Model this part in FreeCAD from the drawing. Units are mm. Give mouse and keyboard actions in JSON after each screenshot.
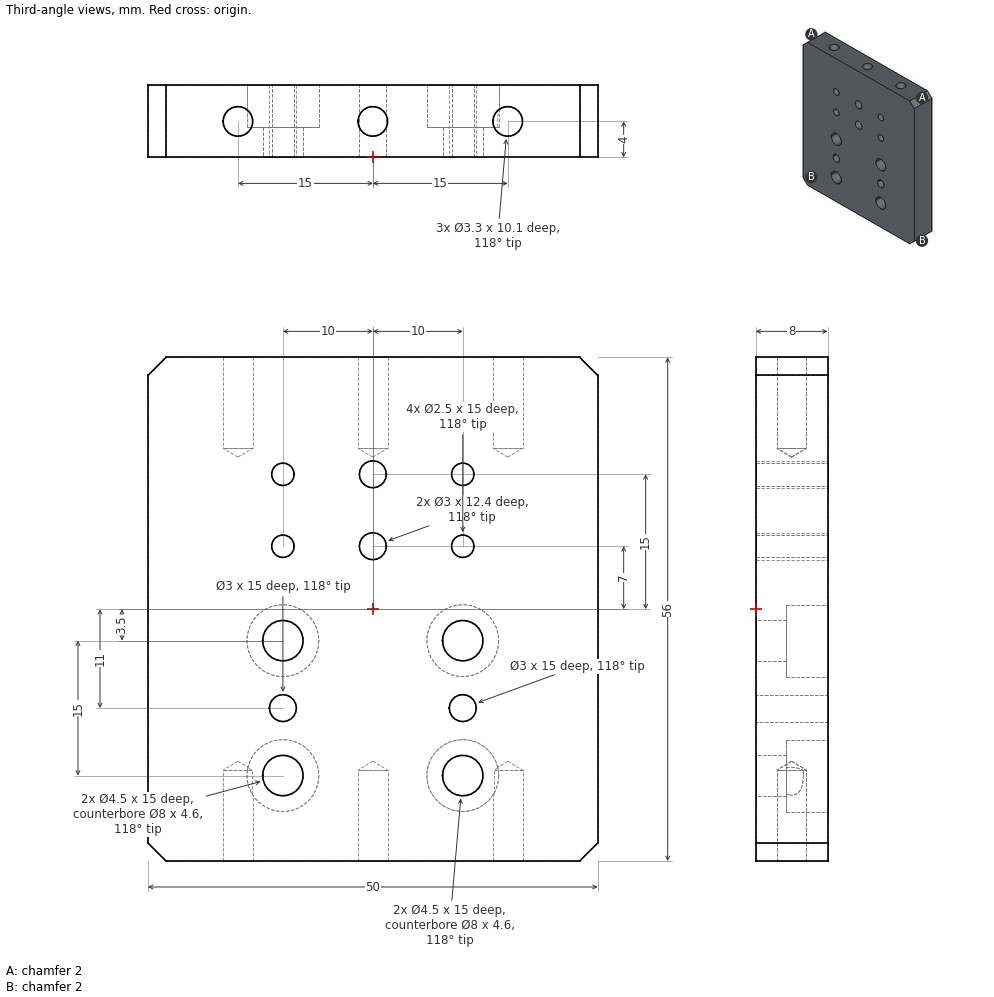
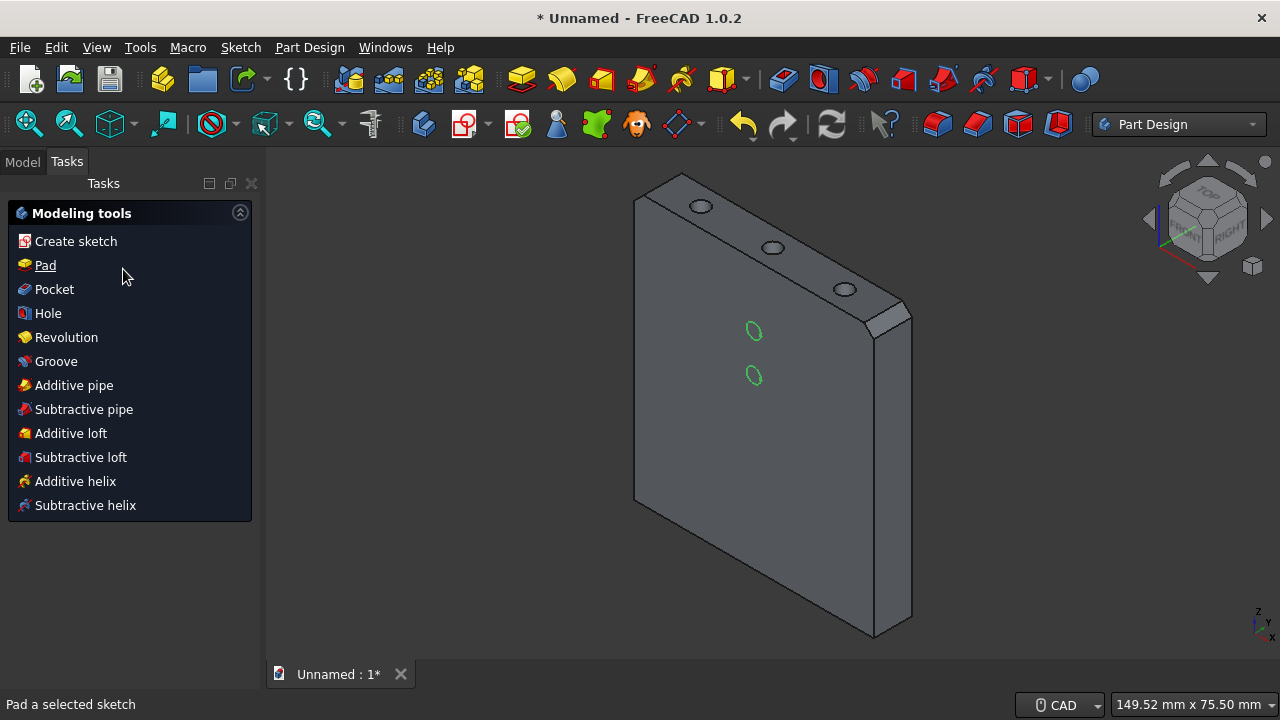
{"action": "left_click", "coordinate": [824, 80]}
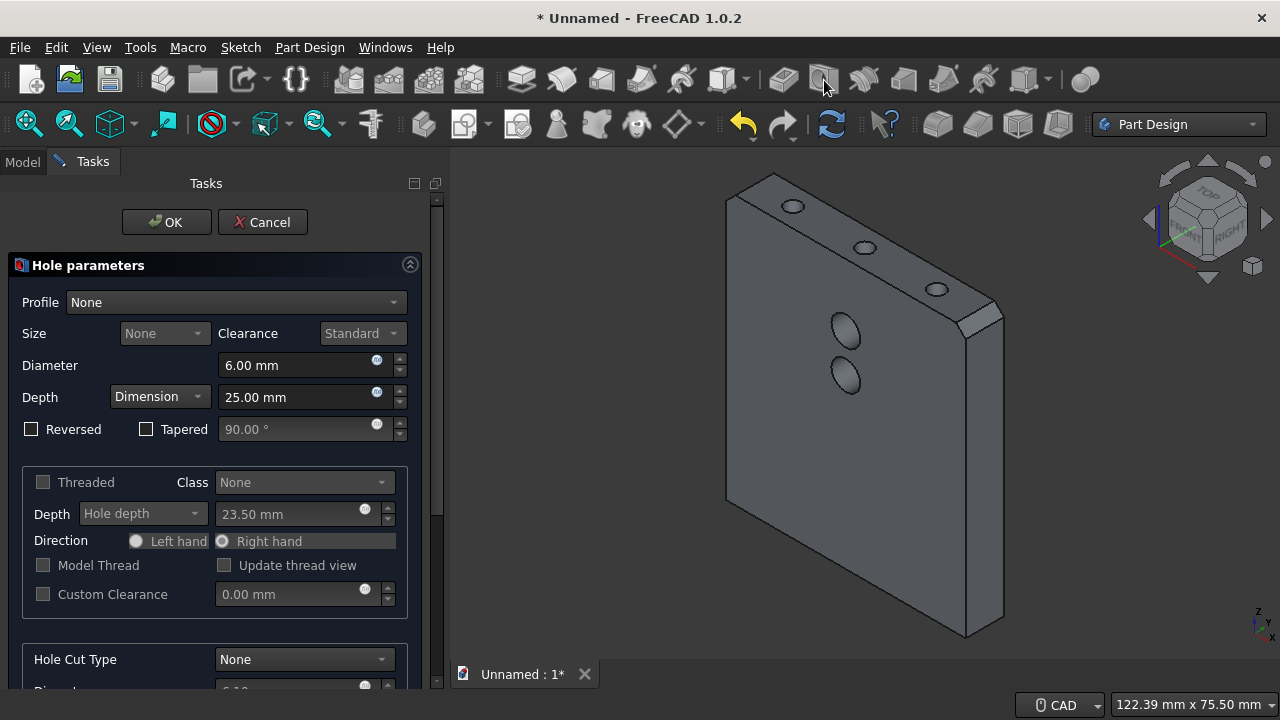
{"action": "triple_click", "coordinate": [305, 365]}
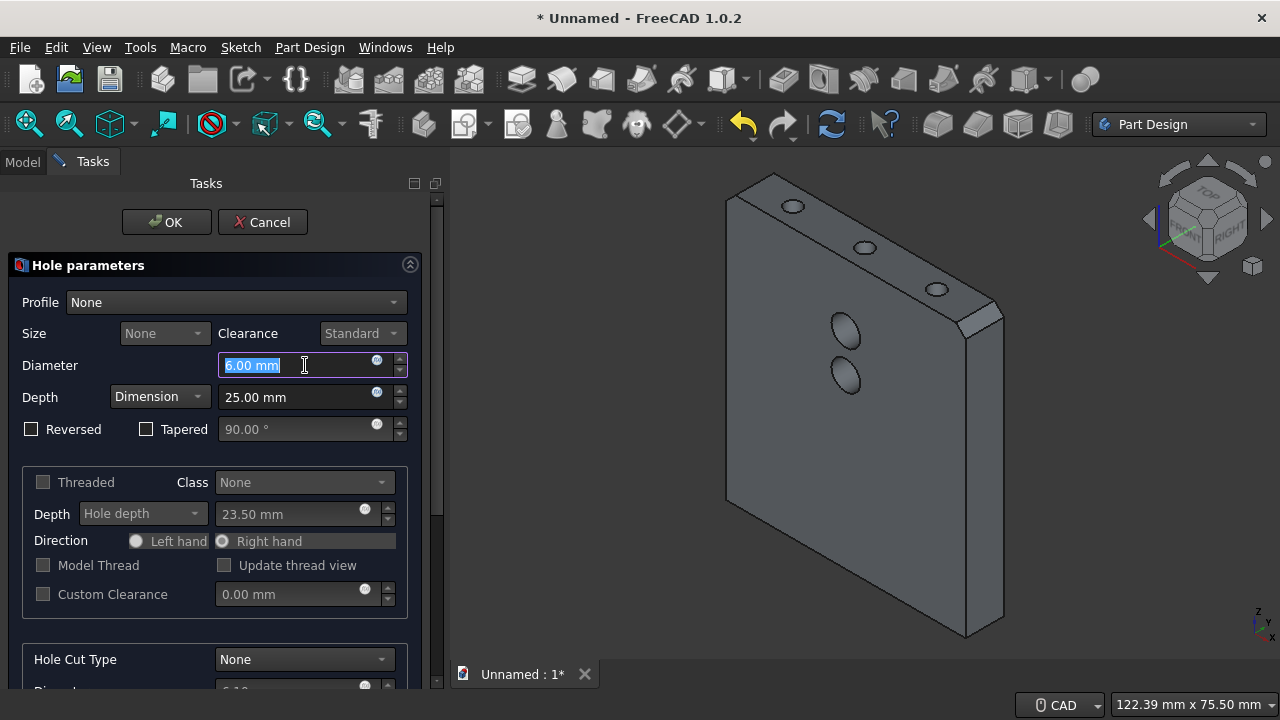
{"action": "type", "text": "3"}
{"action": "key", "text": "Tab"}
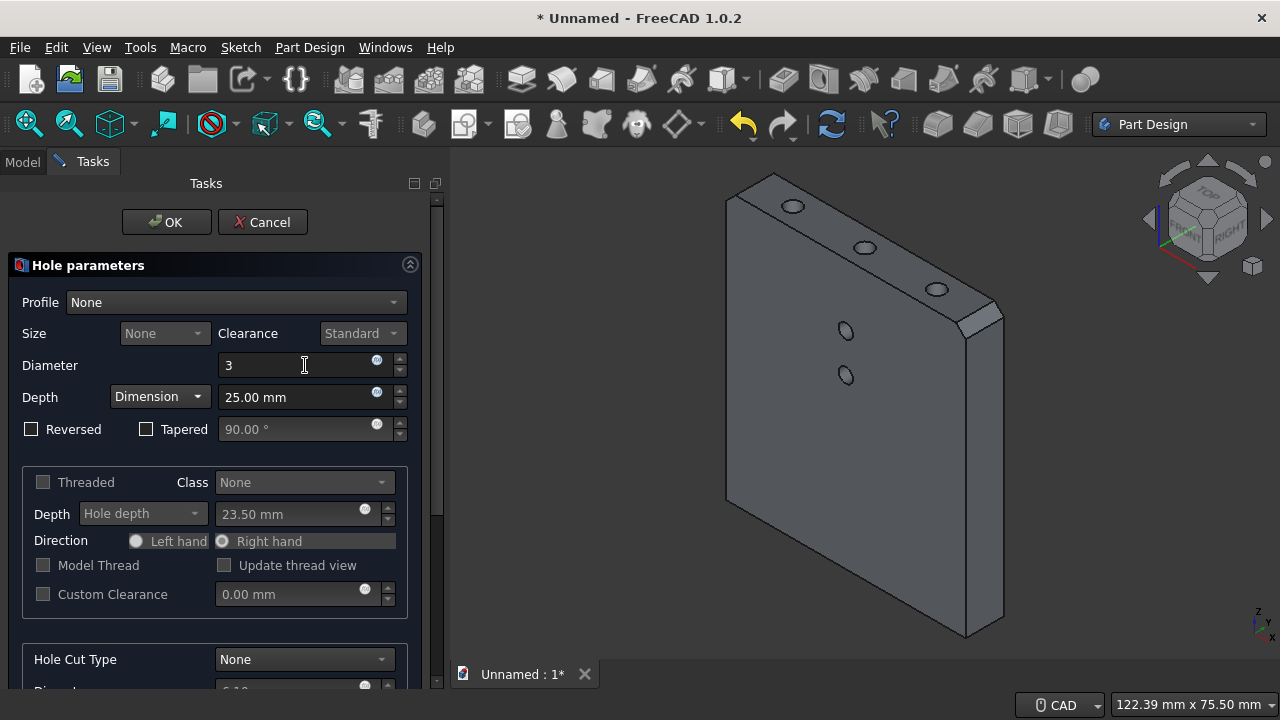
{"action": "triple_click", "coordinate": [305, 397]}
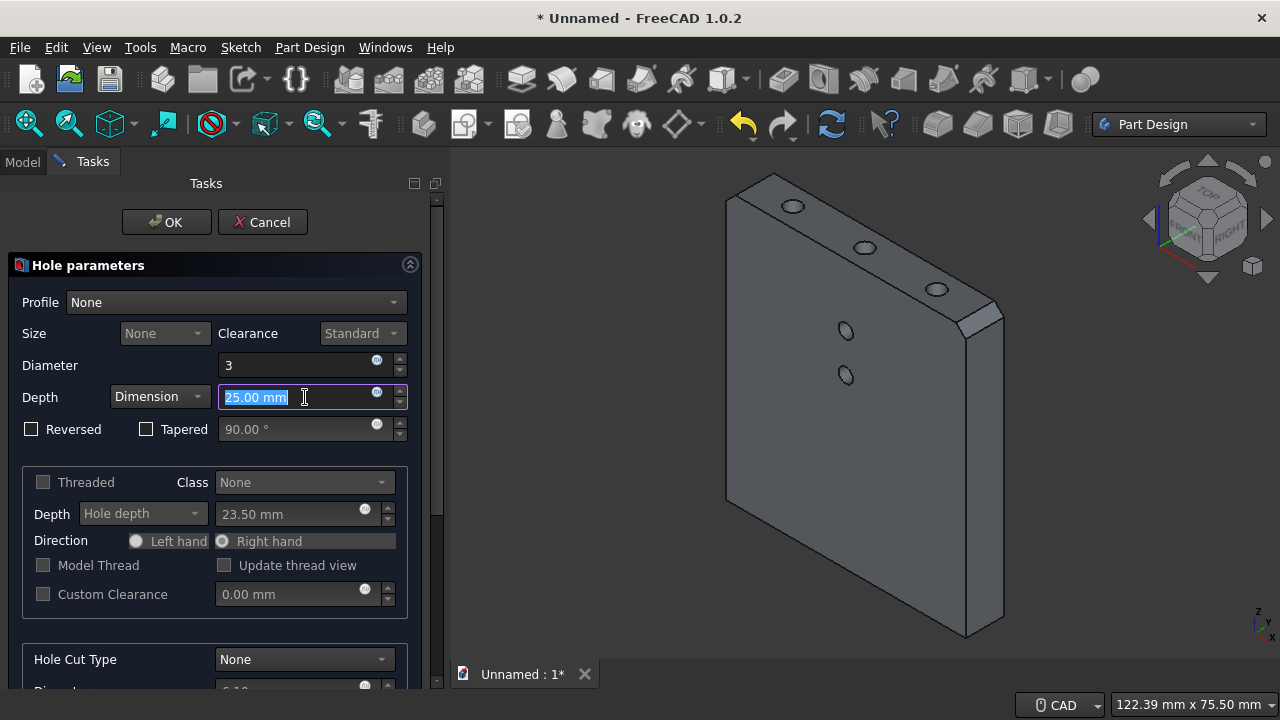
{"action": "type", "text": "12.4"}
{"action": "key", "text": "Tab"}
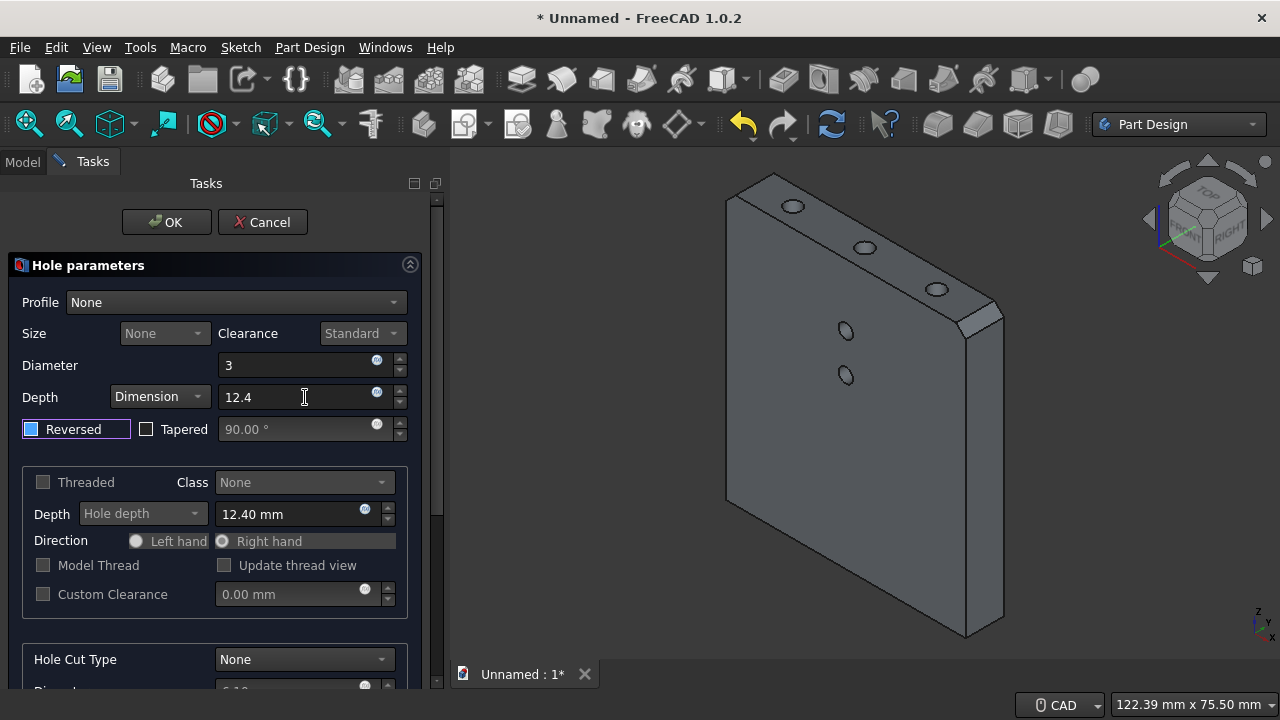
{"action": "left_click", "coordinate": [167, 222]}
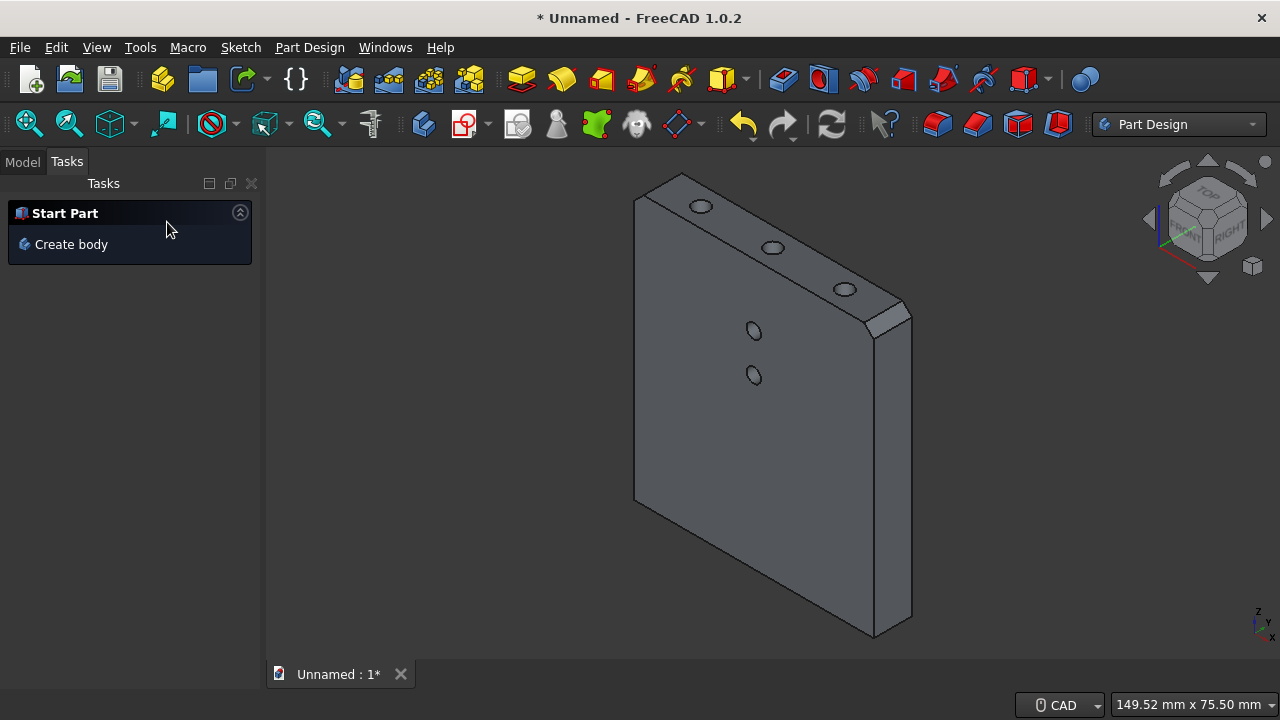
{"action": "left_click", "coordinate": [788, 477]}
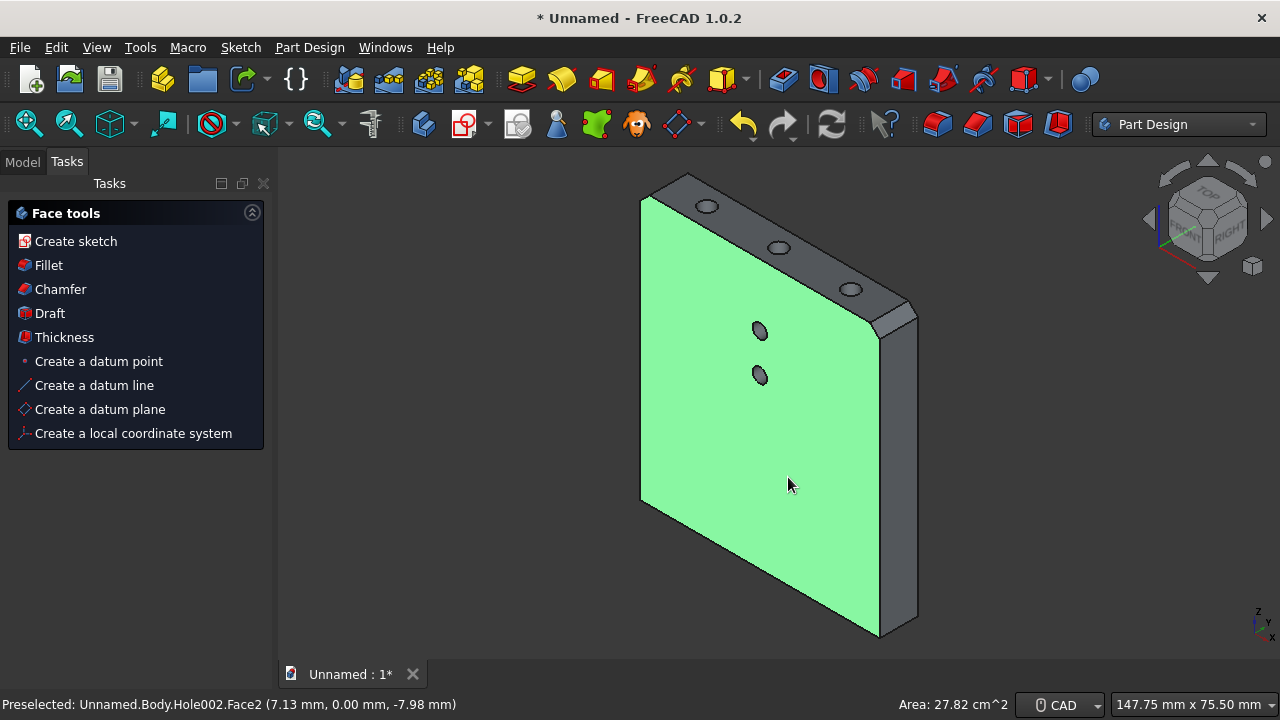
{"action": "left_click", "coordinate": [464, 124]}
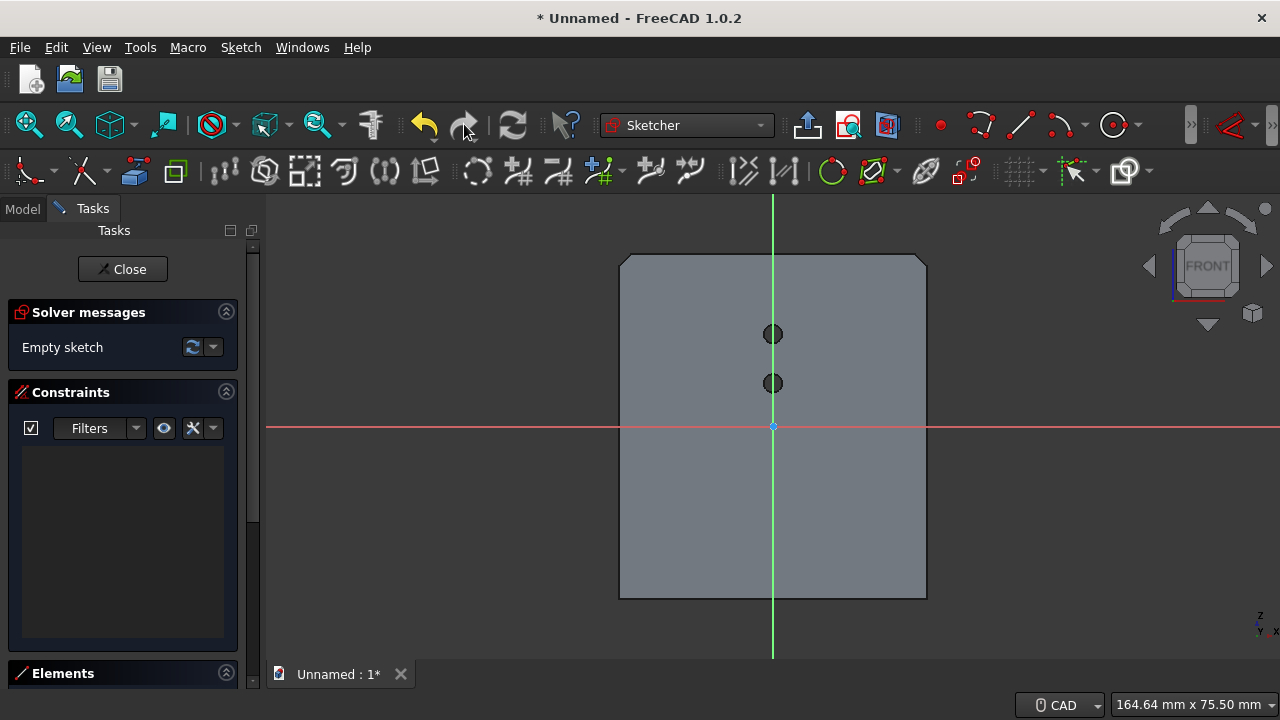
{"action": "scroll", "coordinate": [813, 347], "scroll_direction": "up", "scroll_amount": 5}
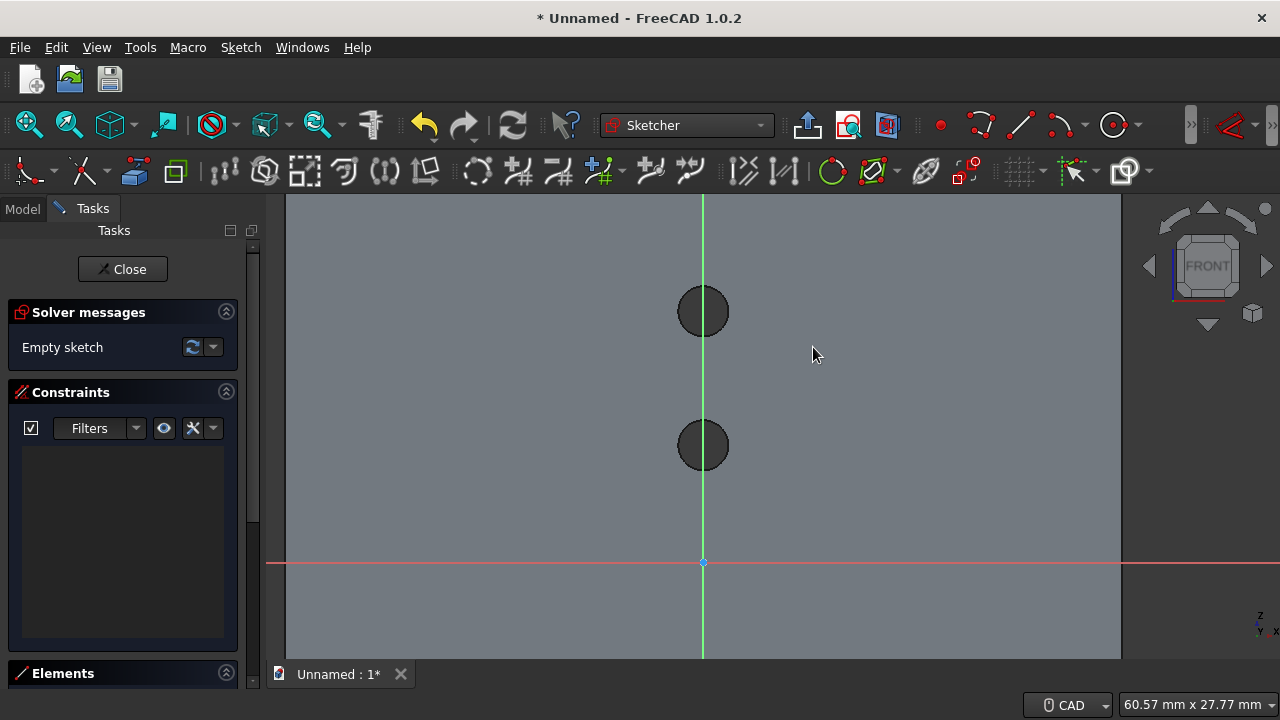
{"action": "left_click", "coordinate": [1114, 126]}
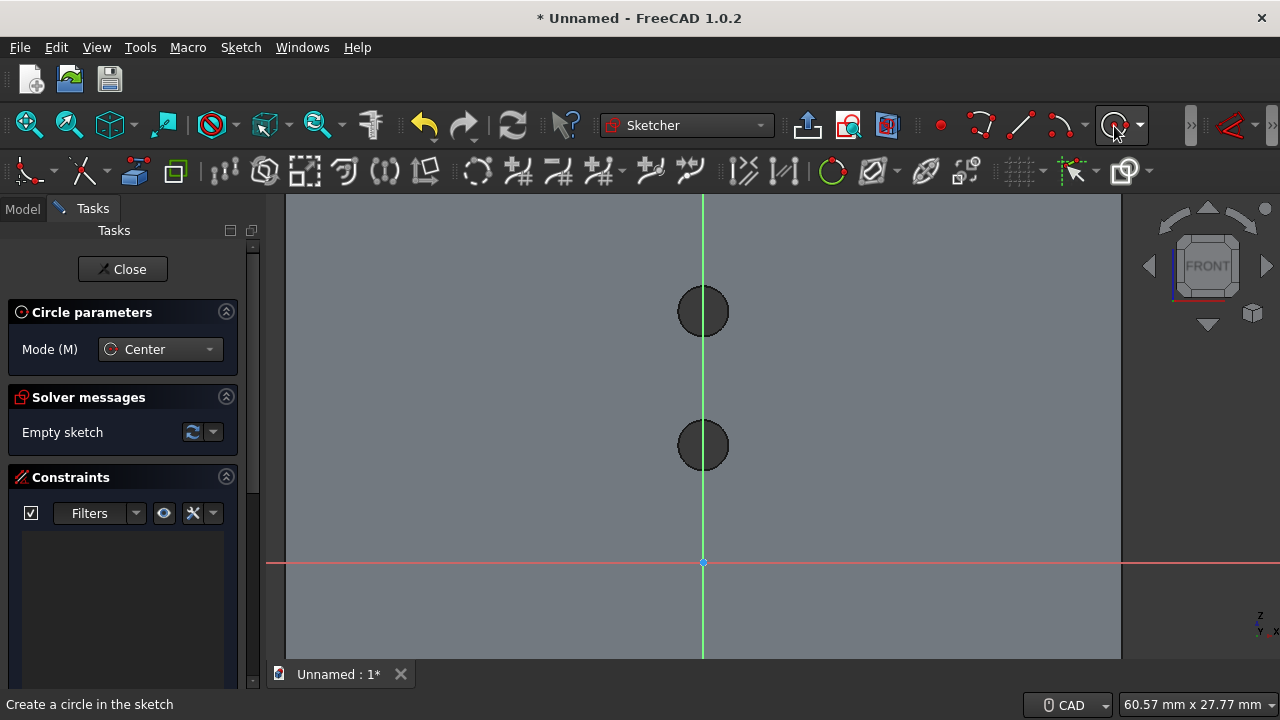
{"action": "left_click", "coordinate": [871, 445]}
{"action": "mouse_move", "coordinate": [886, 431]}